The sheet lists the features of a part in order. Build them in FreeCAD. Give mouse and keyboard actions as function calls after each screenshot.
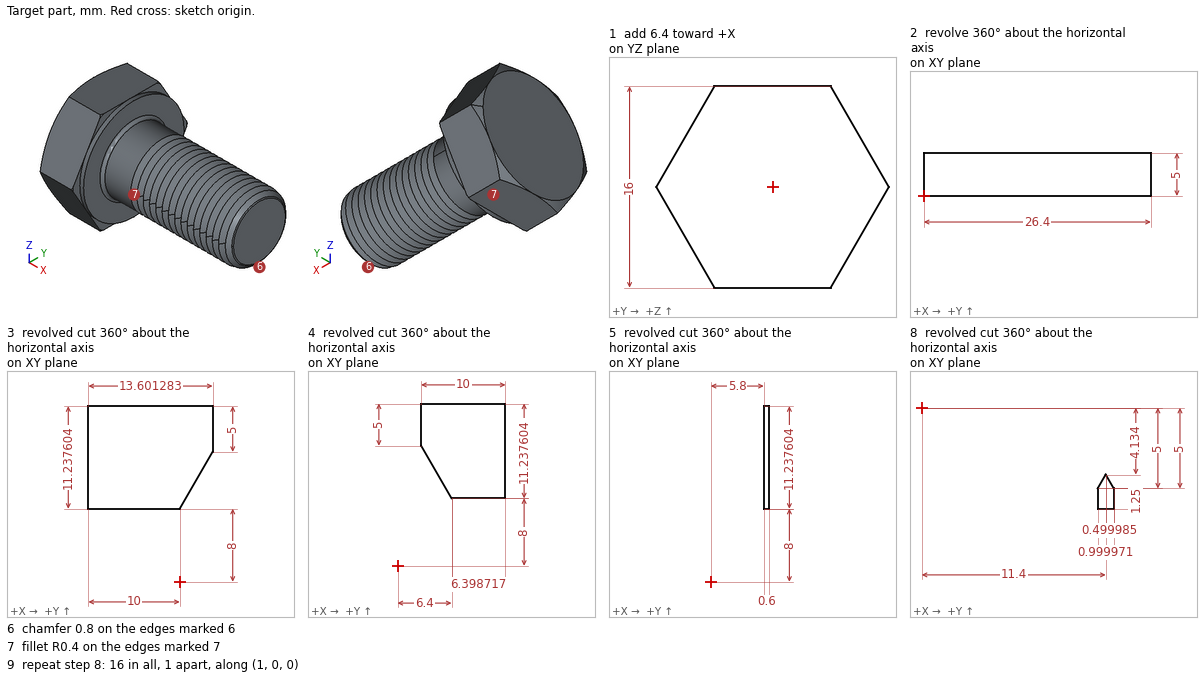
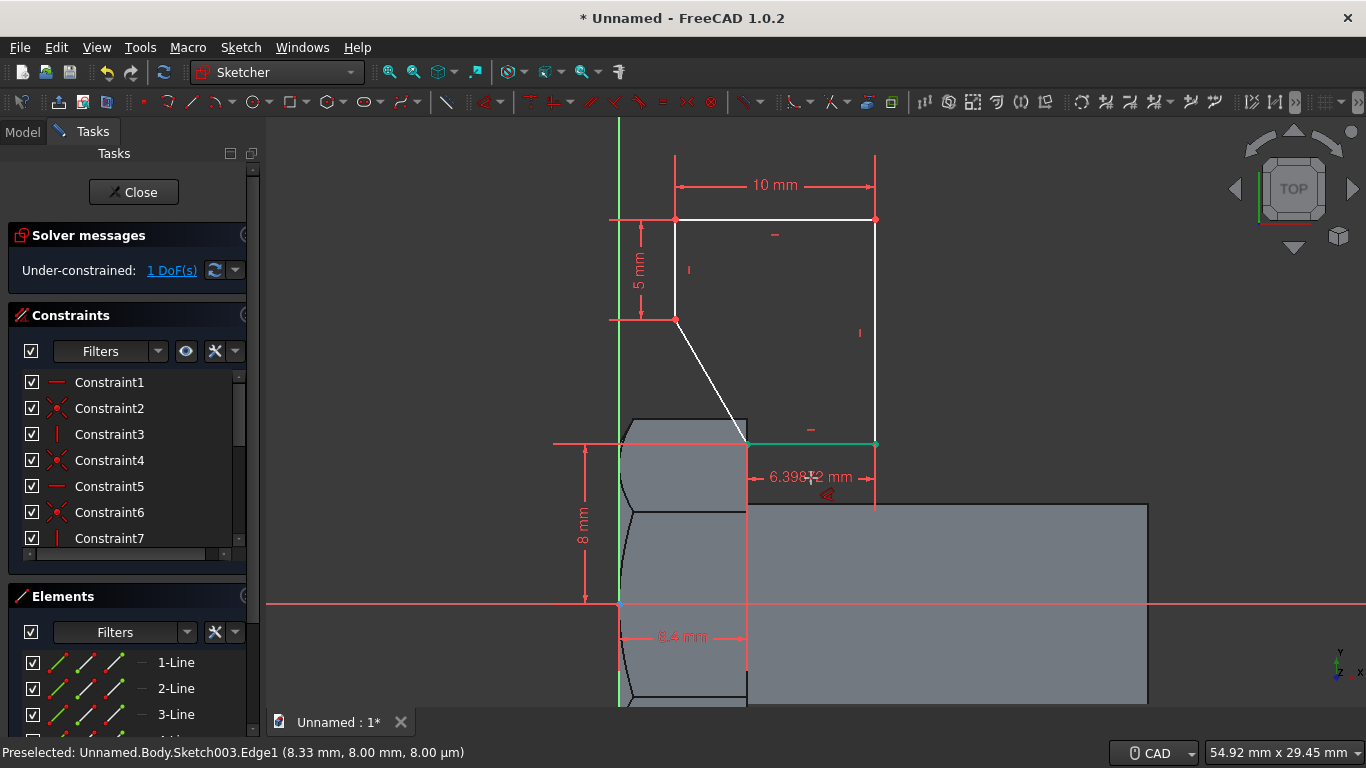
click(875, 377)
click(909, 332)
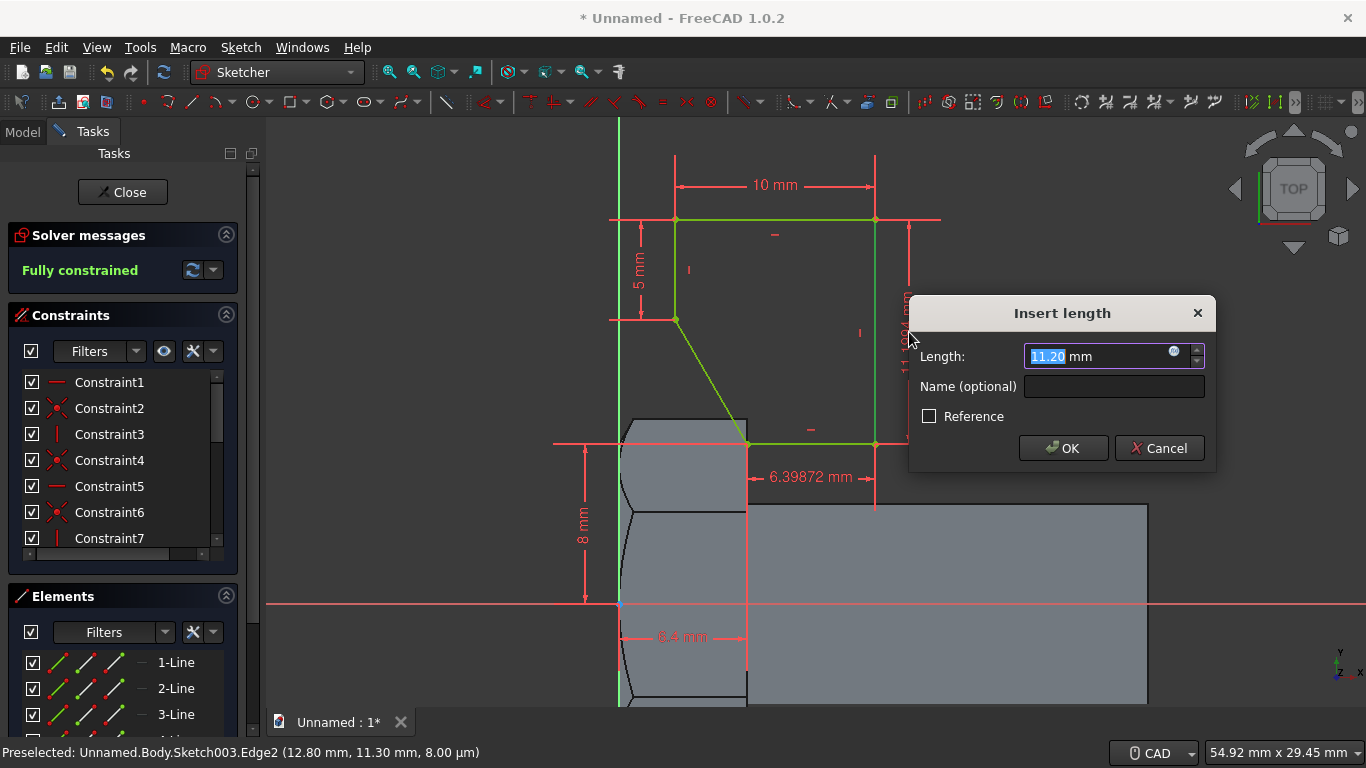
text(11.237604)
key(Return)
key(Escape)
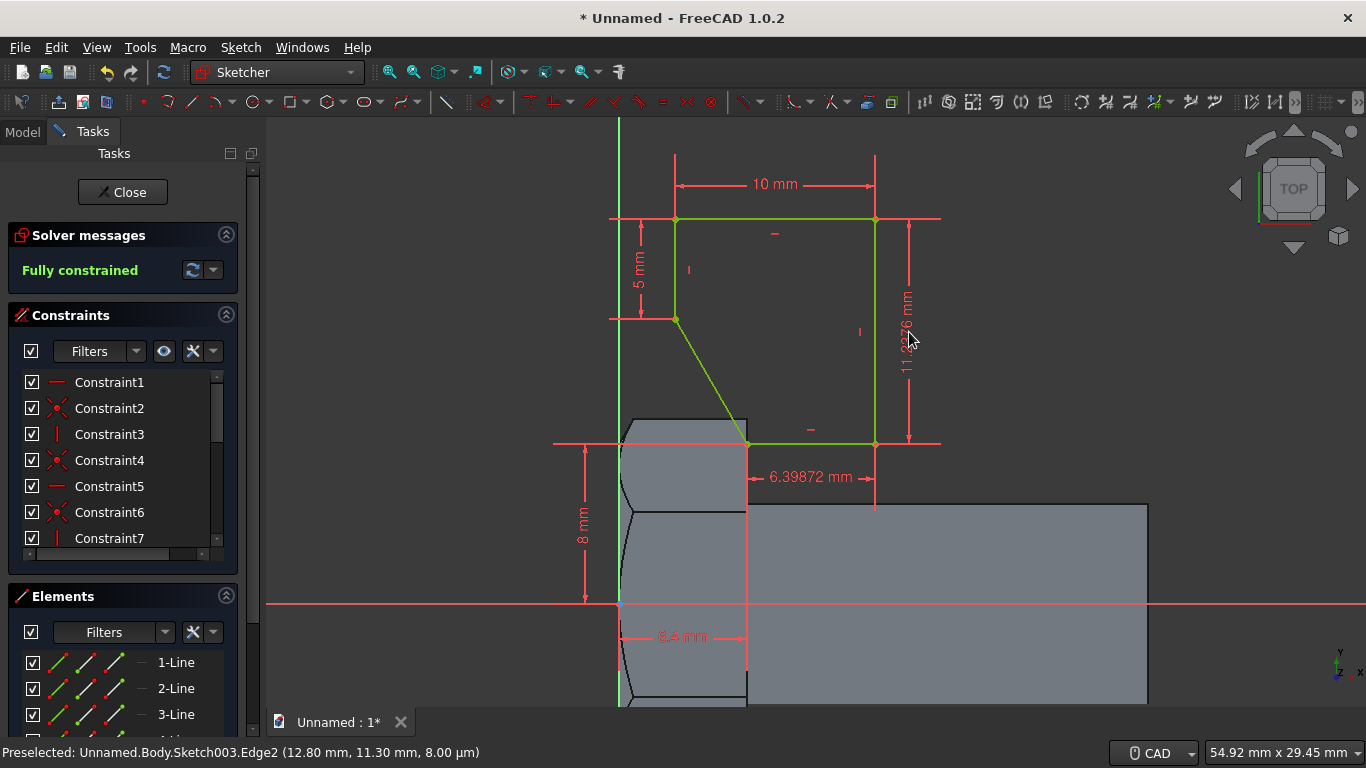
click(123, 192)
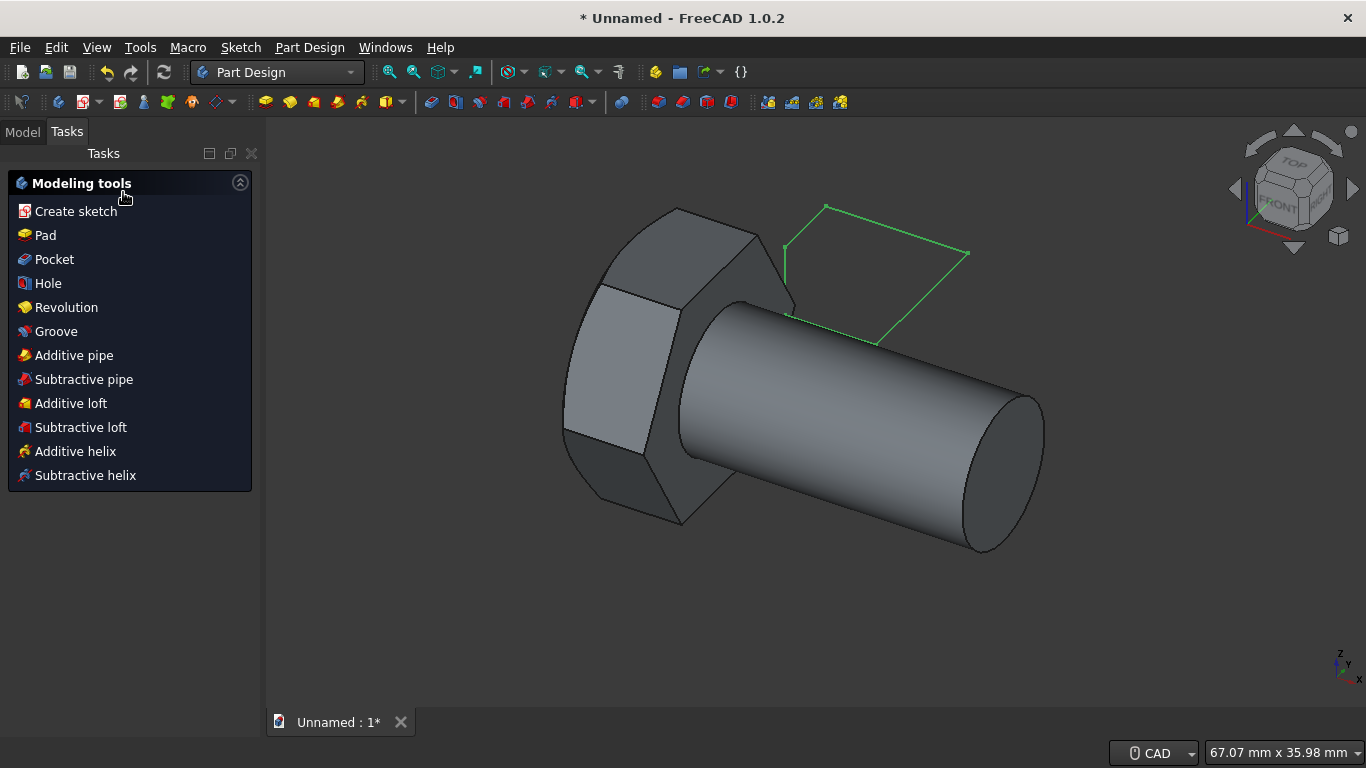
click(480, 102)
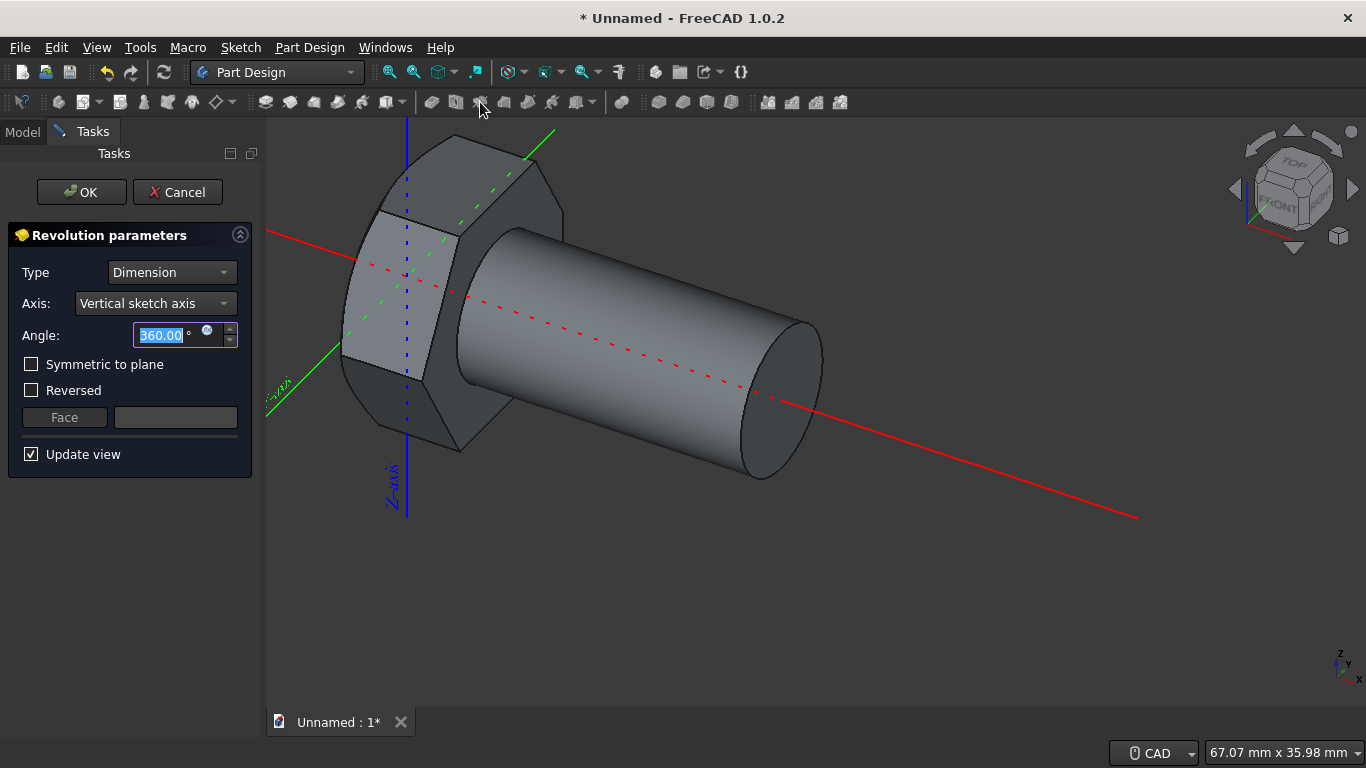
click(156, 304)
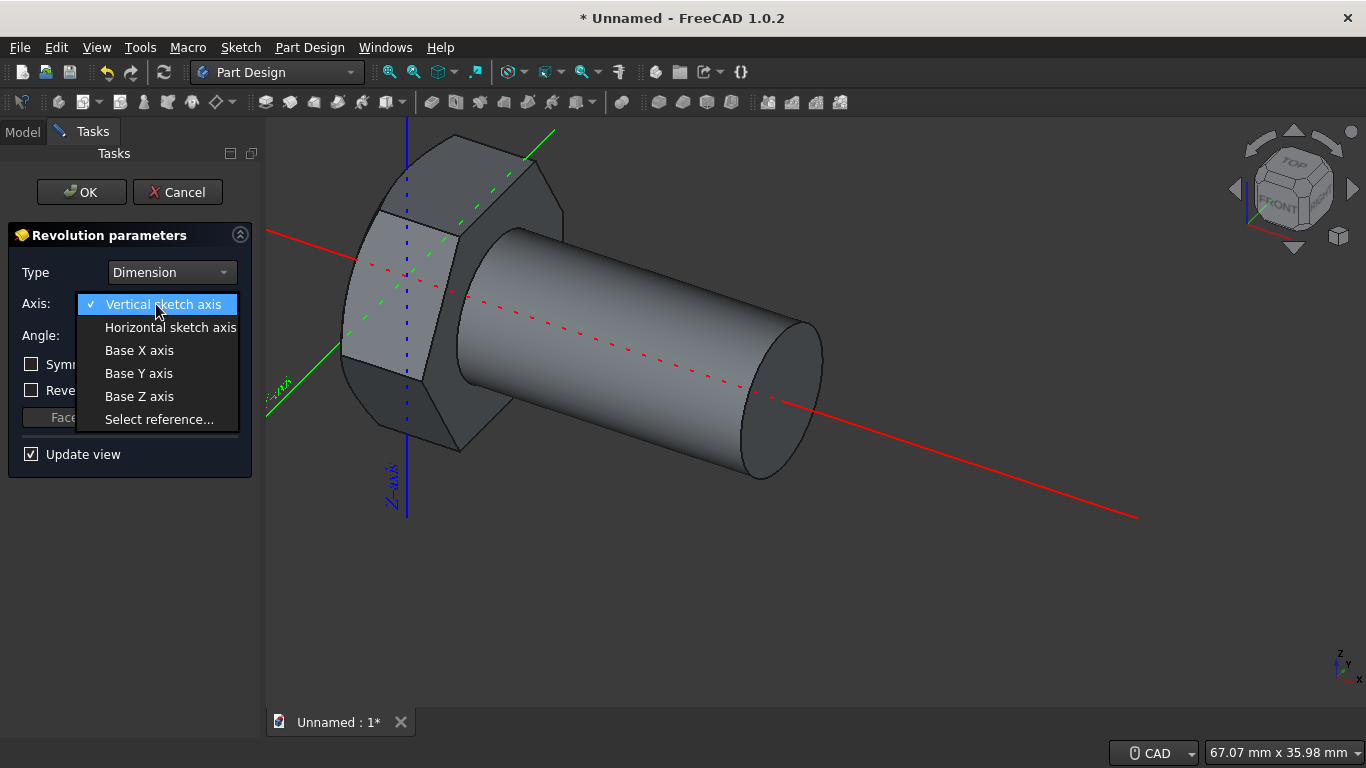
click(156, 328)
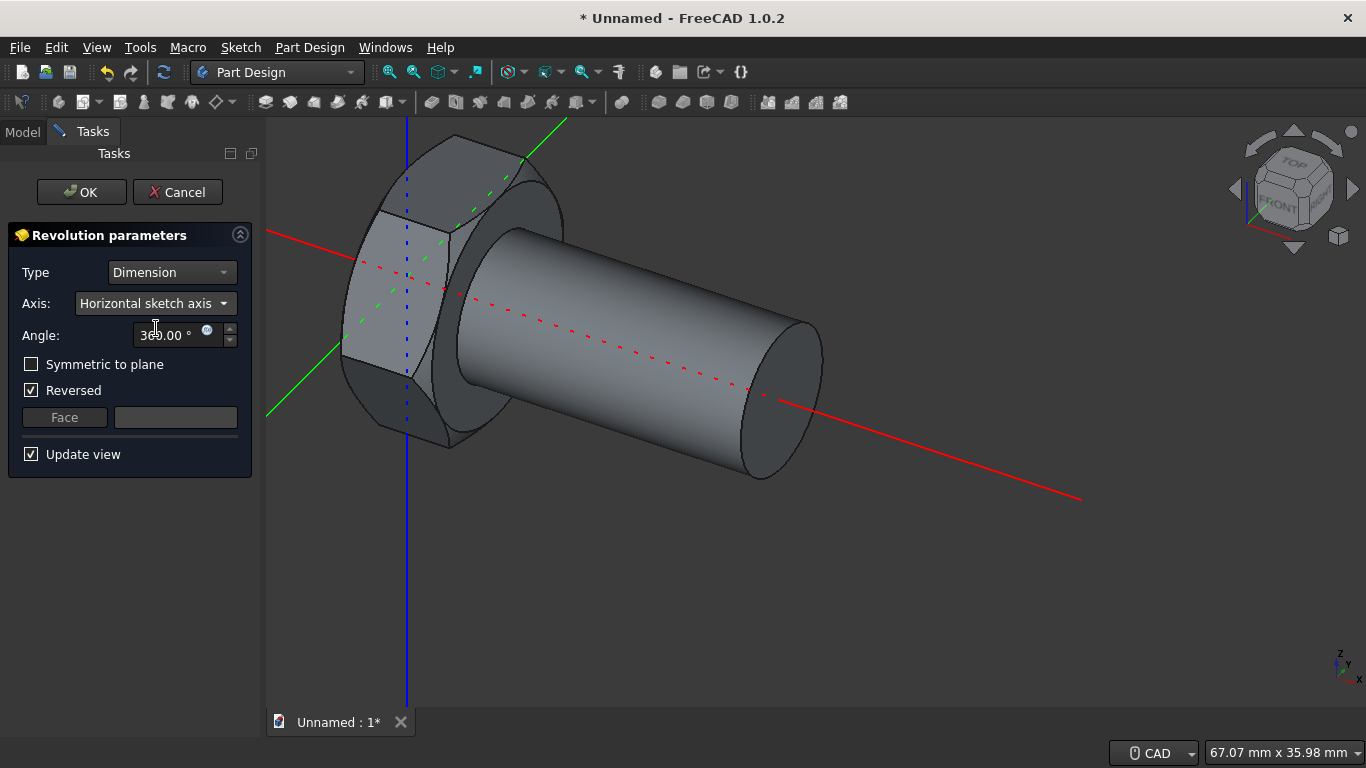
click(82, 192)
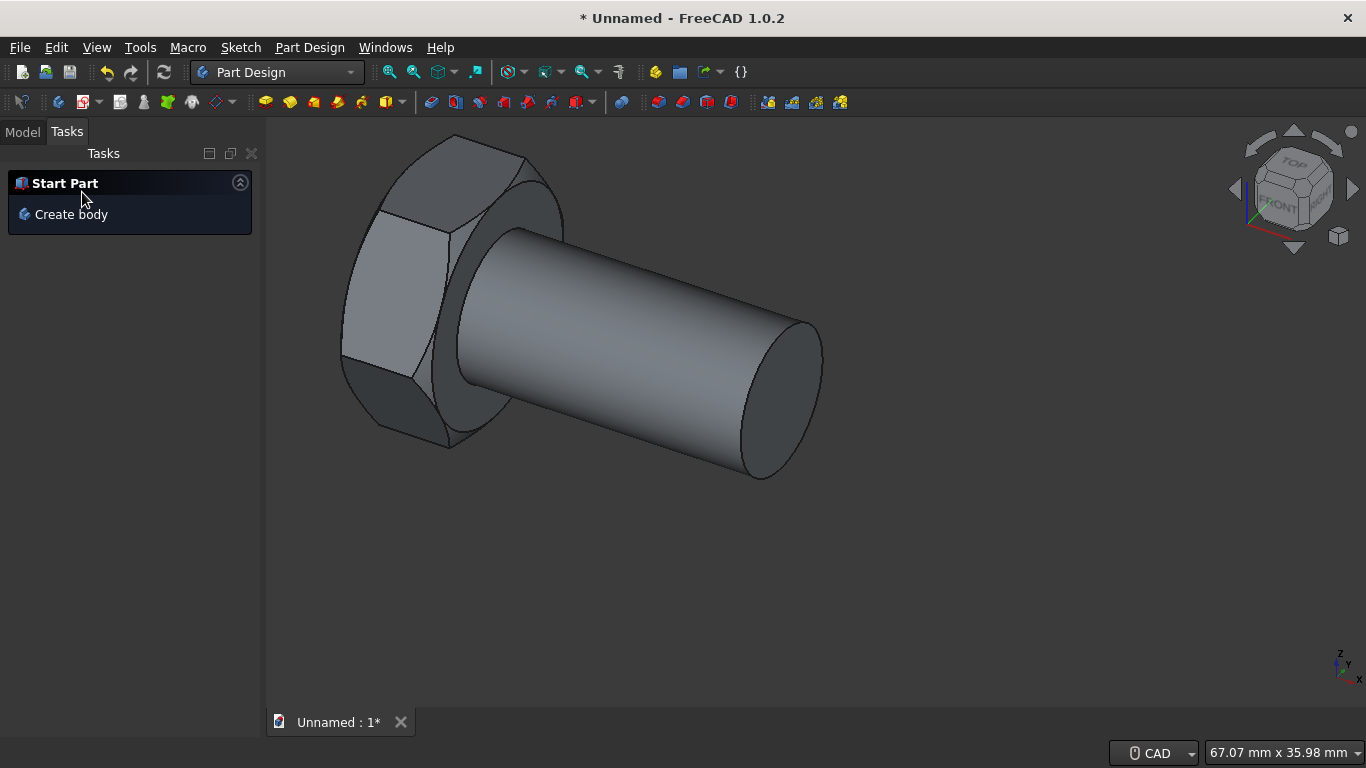
key(v)
key(f)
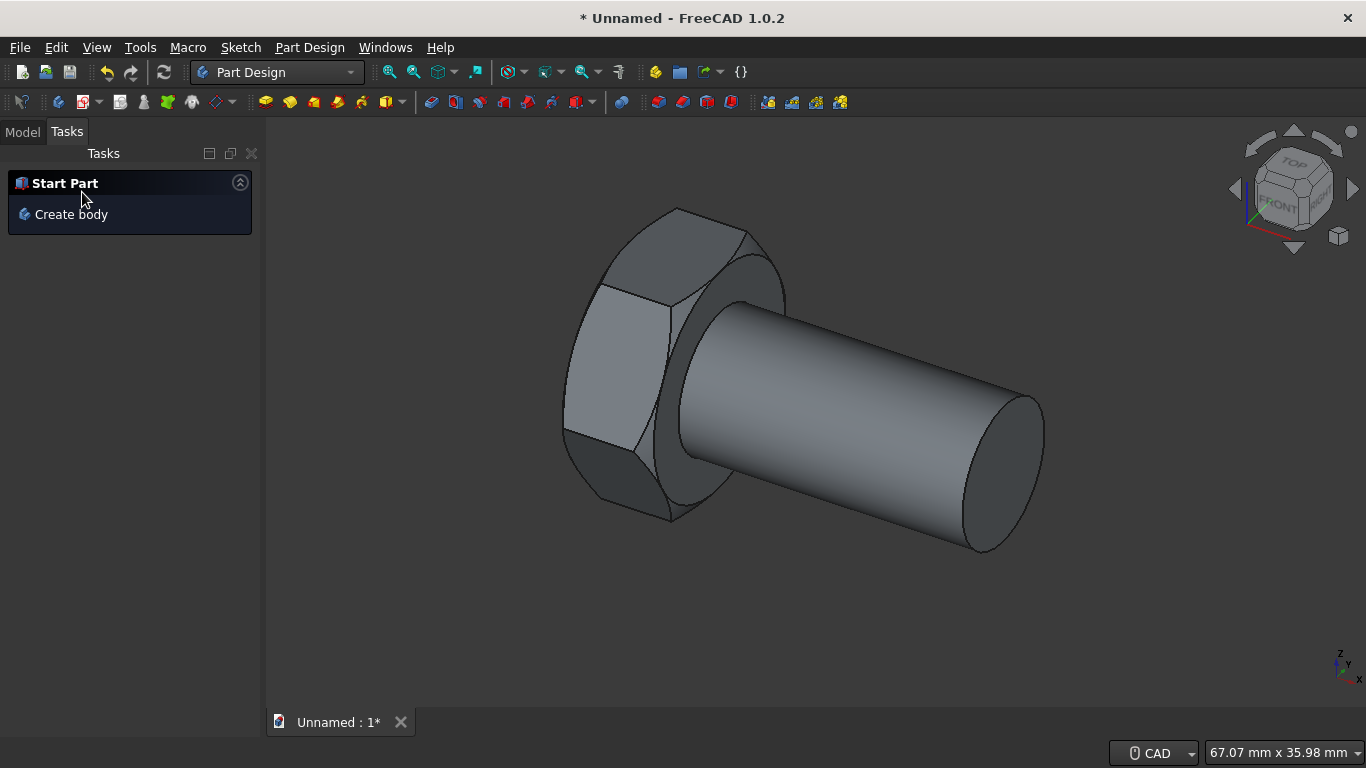
click(84, 102)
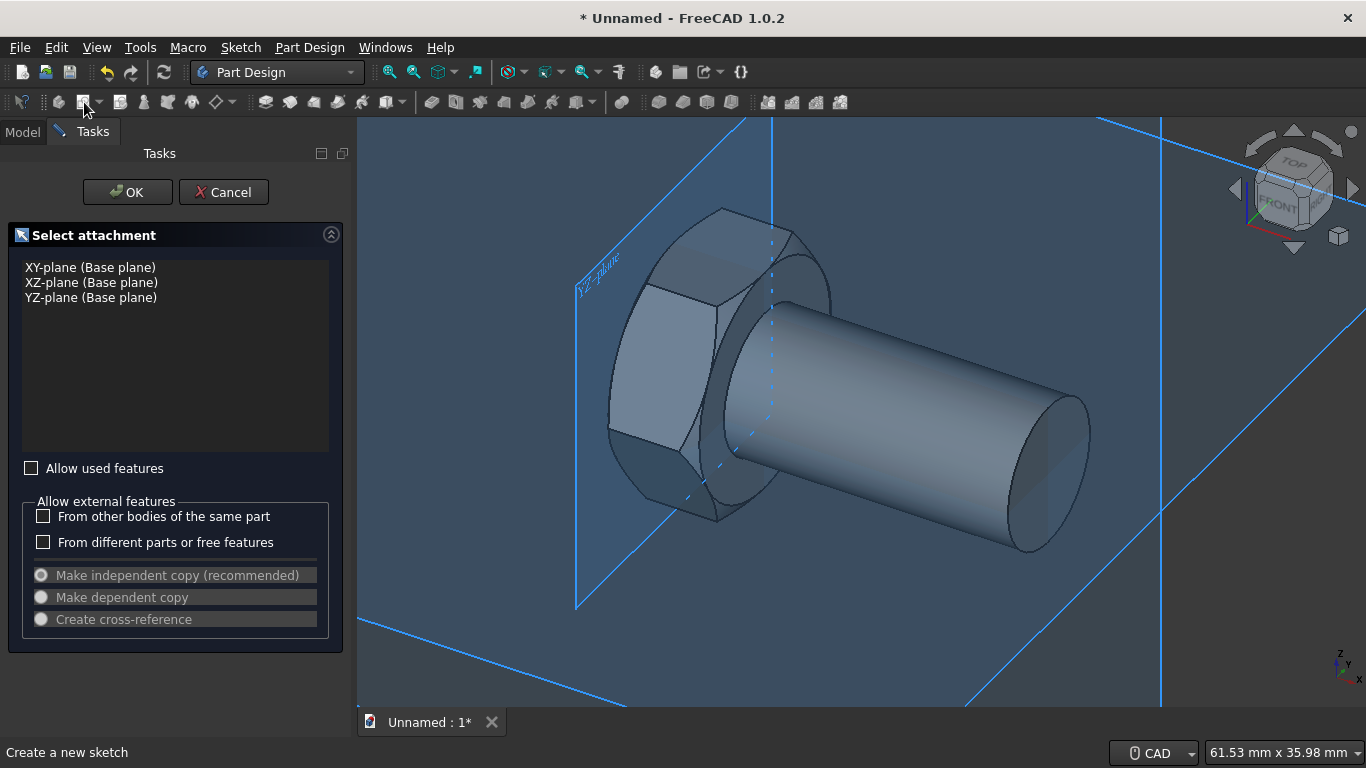
click(82, 268)